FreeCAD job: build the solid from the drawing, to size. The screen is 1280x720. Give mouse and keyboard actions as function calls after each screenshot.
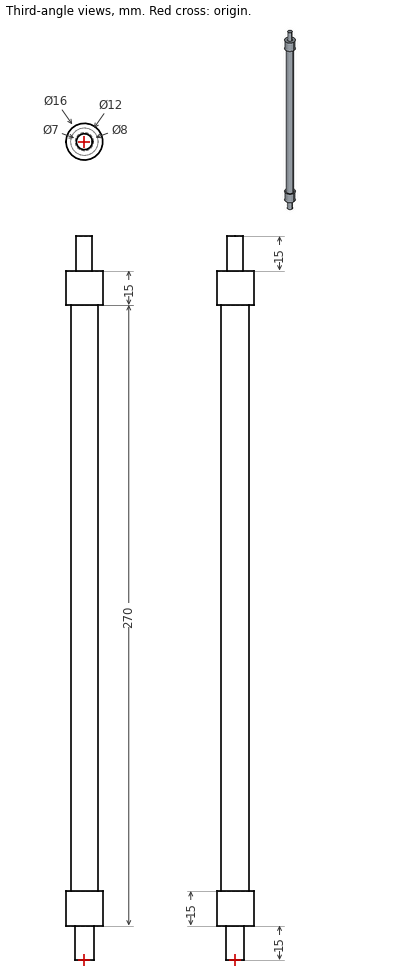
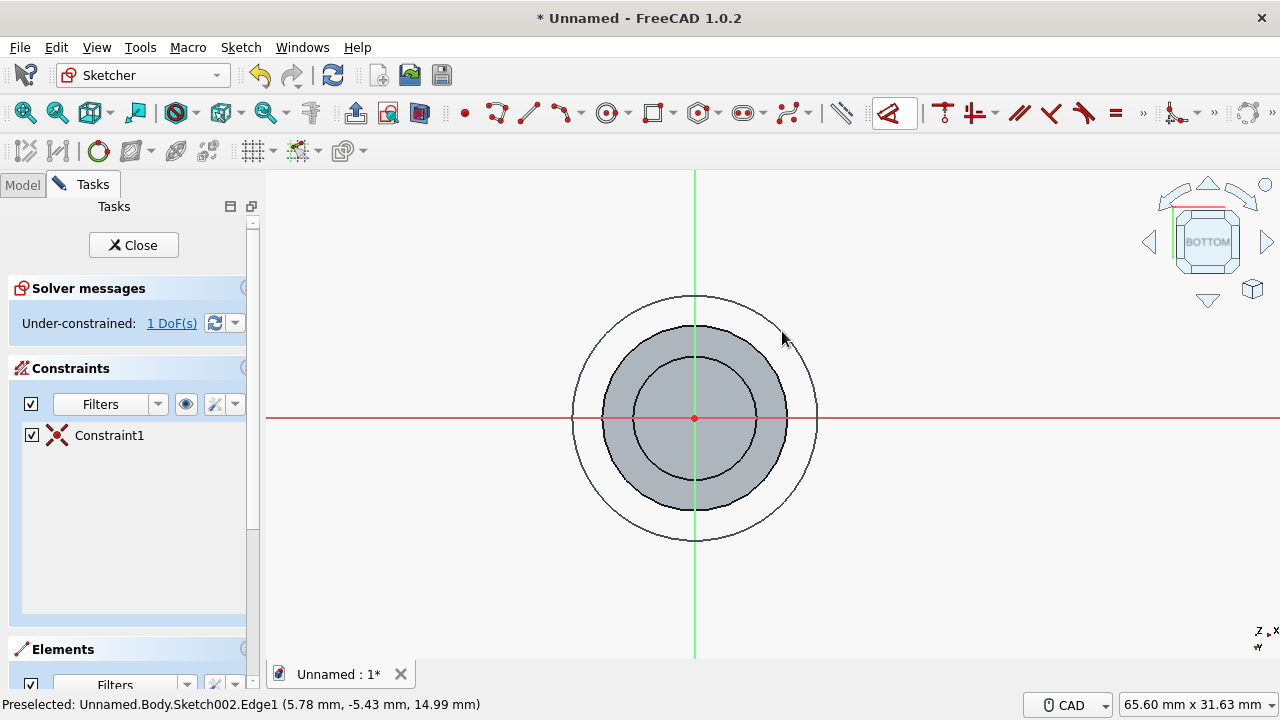
click(781, 331)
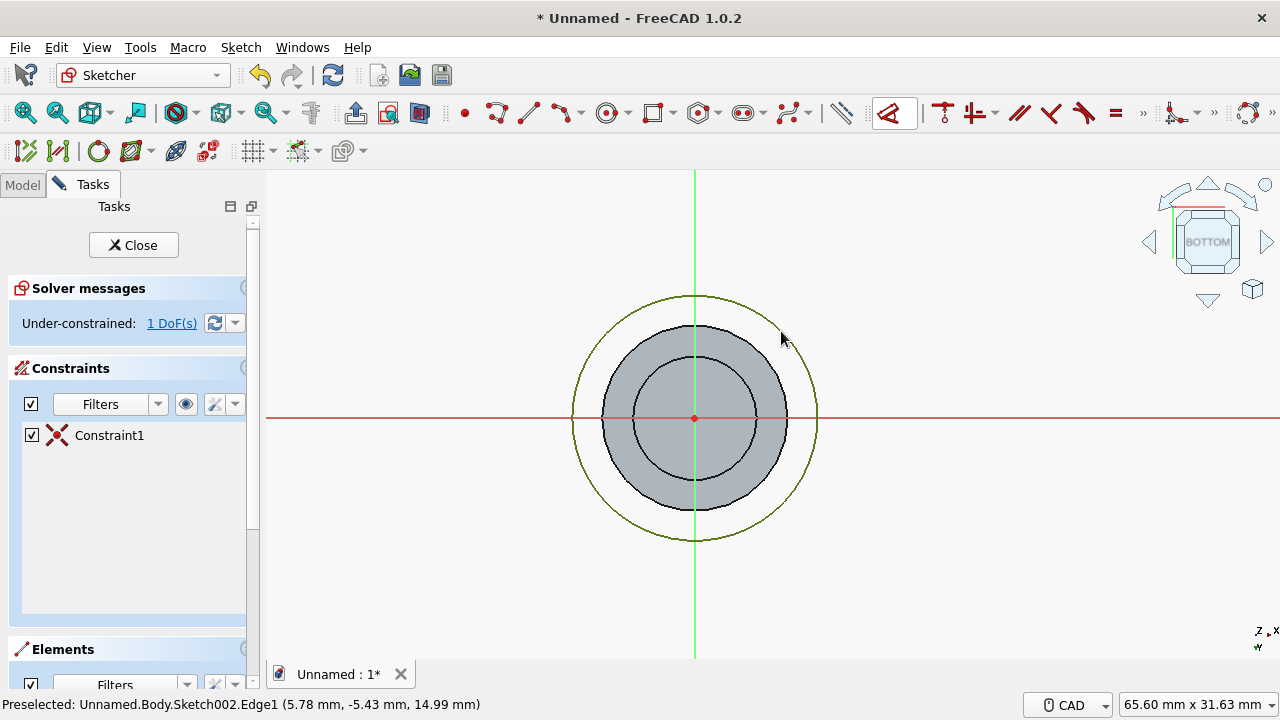
click(912, 114)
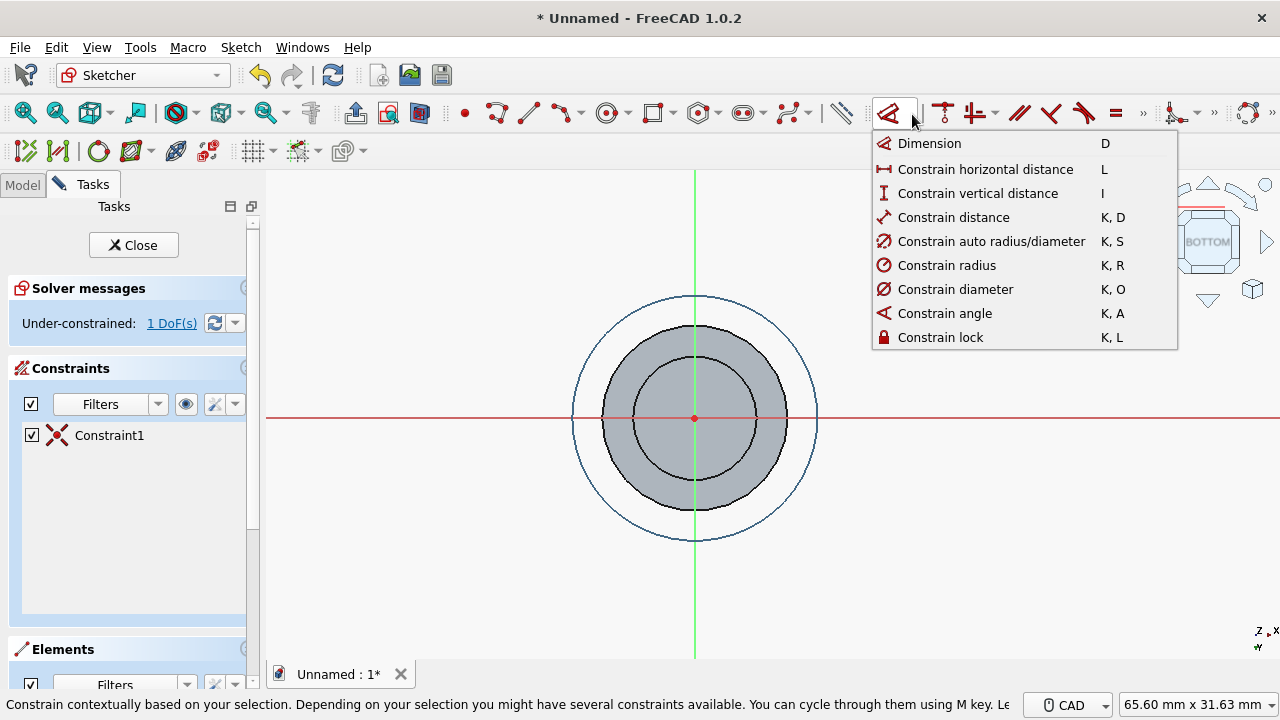
click(1025, 289)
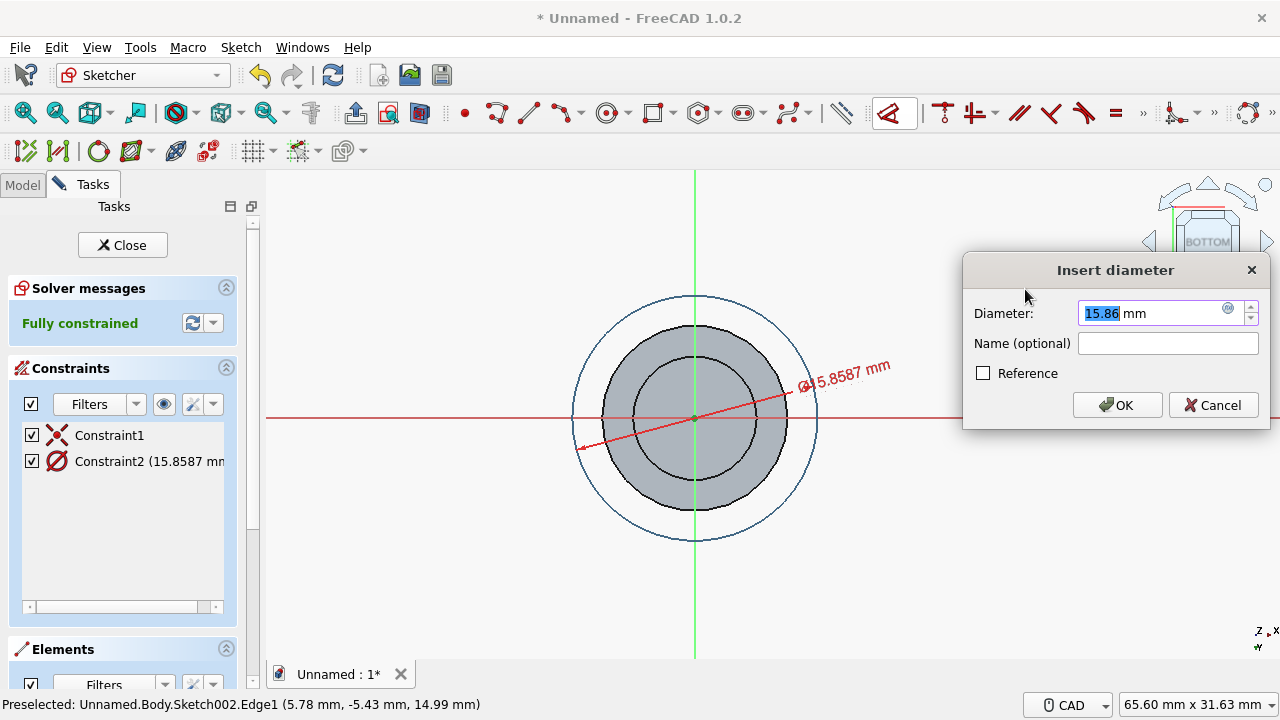
text(16)
key(Return)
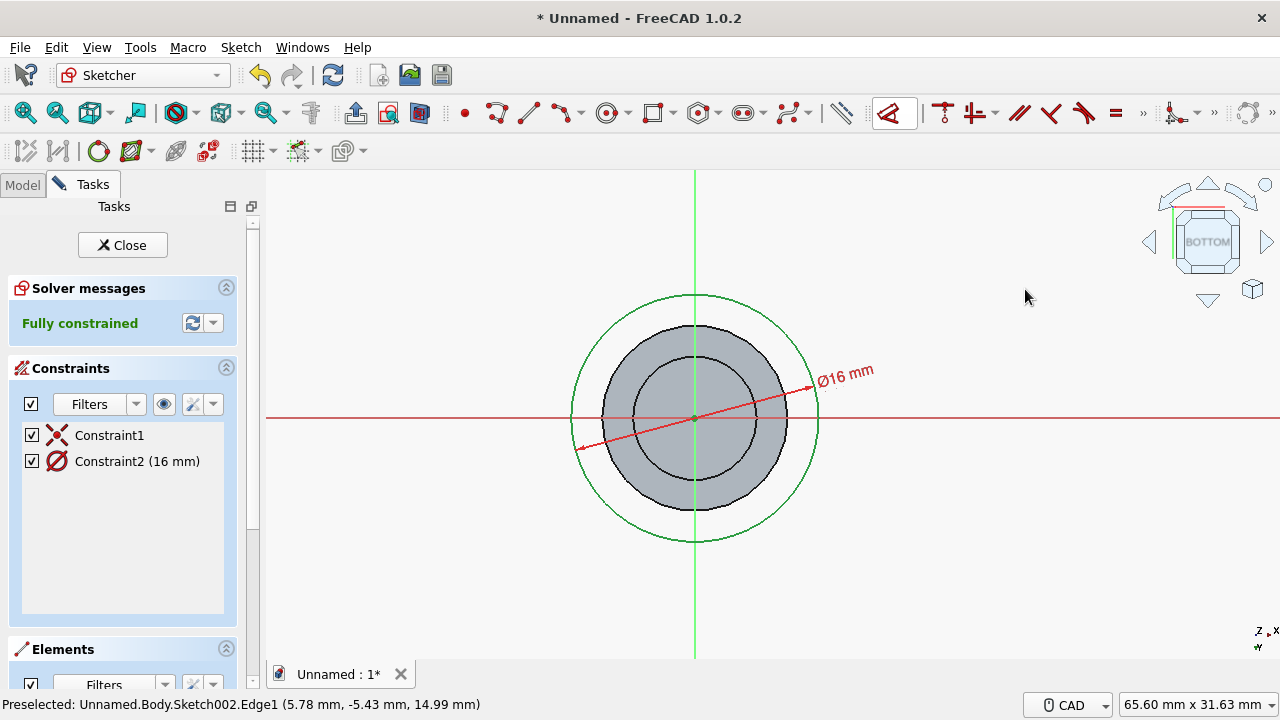
click(123, 245)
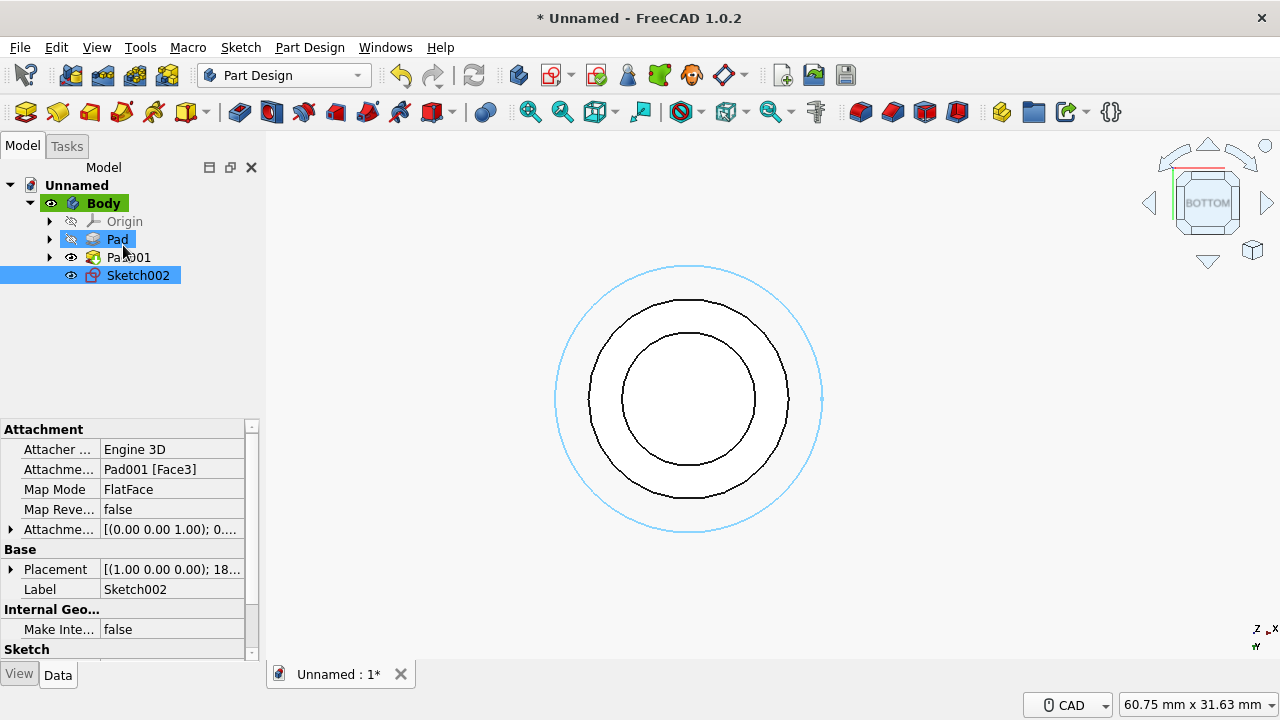
click(26, 112)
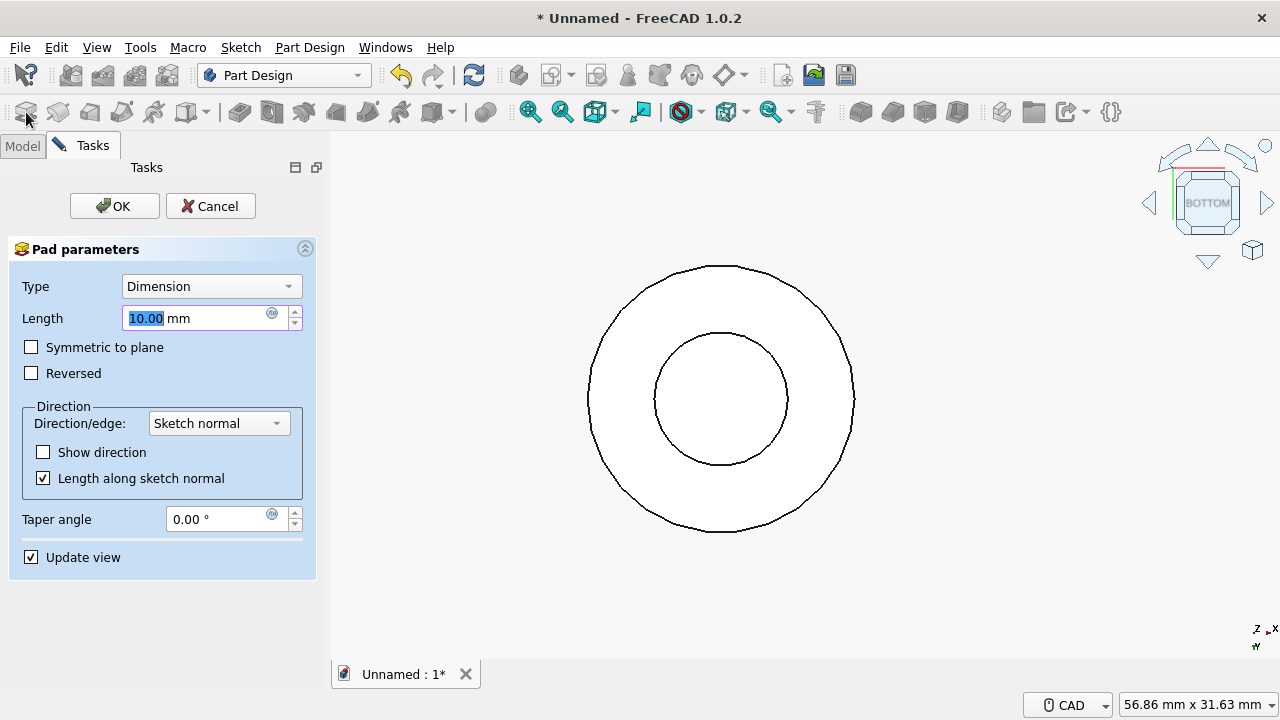
text(15)
key(Tab)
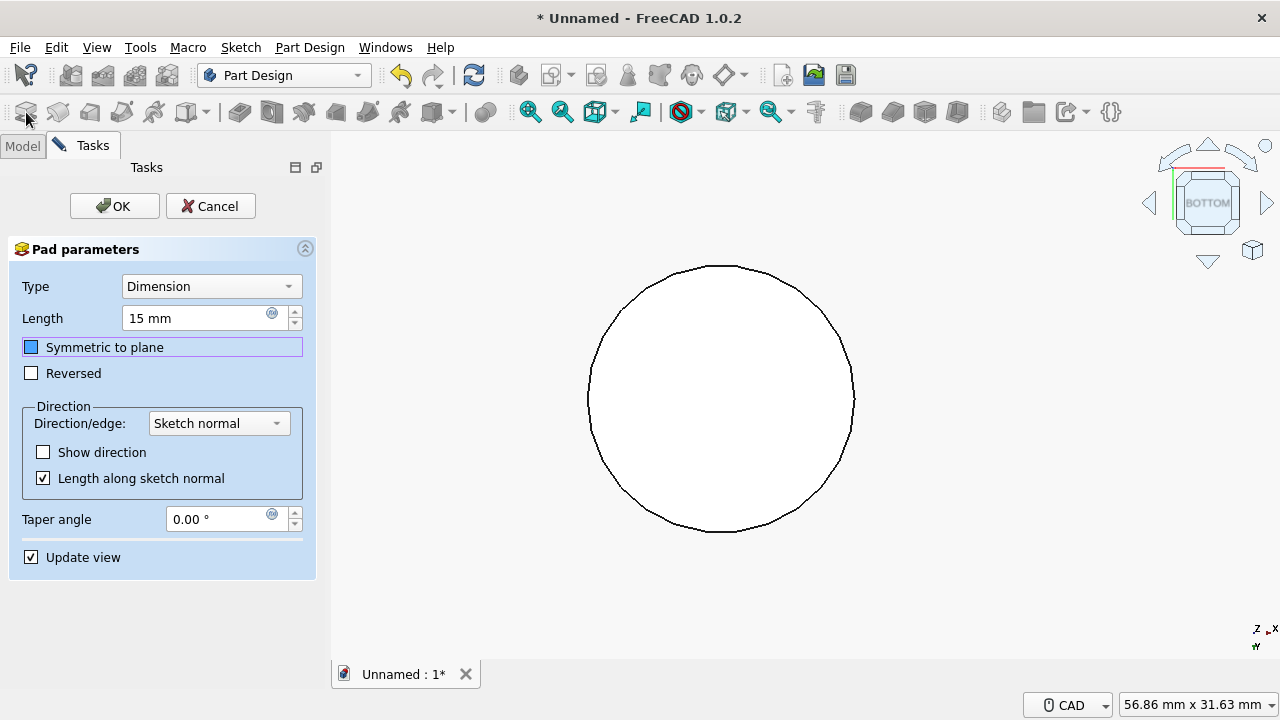
click(30, 373)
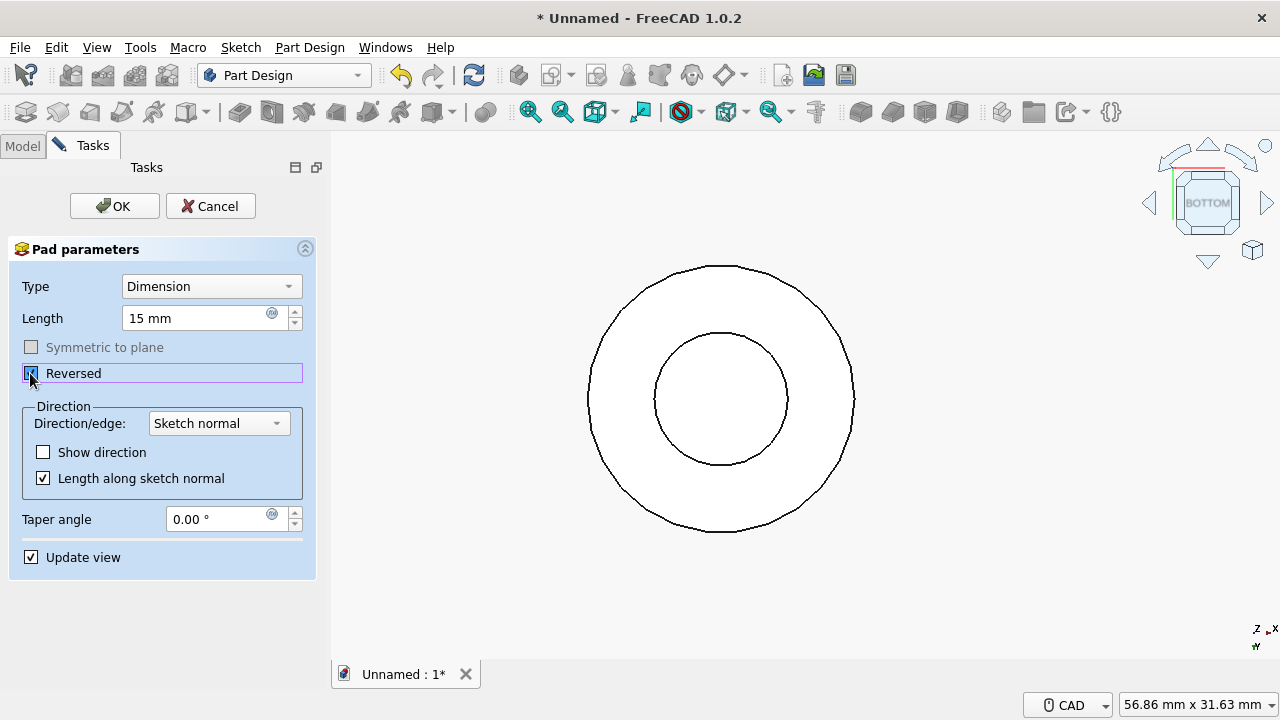
click(115, 206)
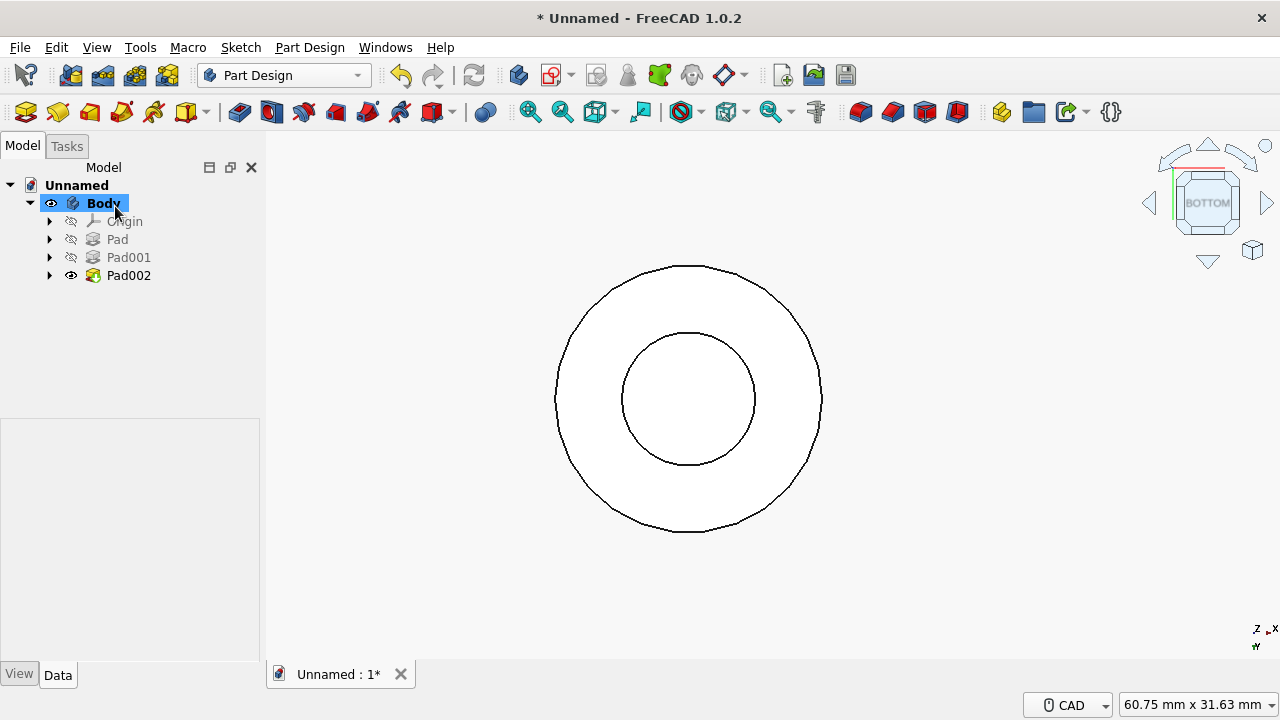
key(0)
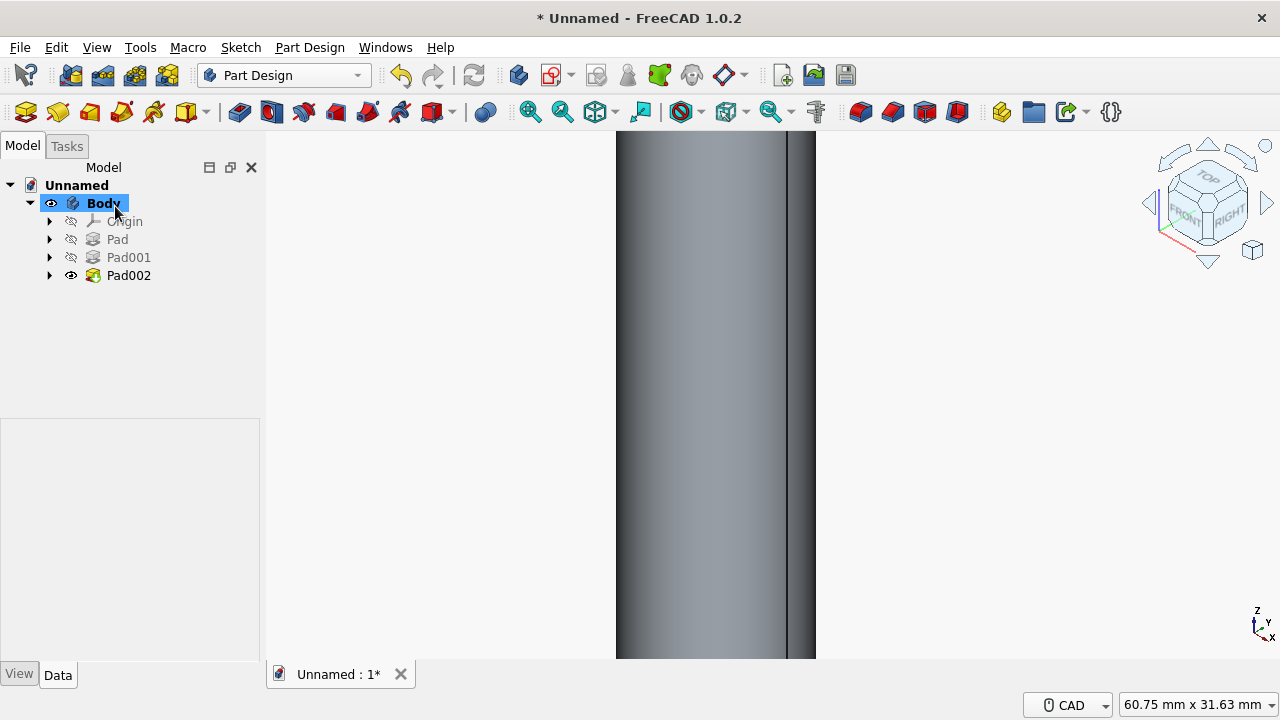
click(532, 112)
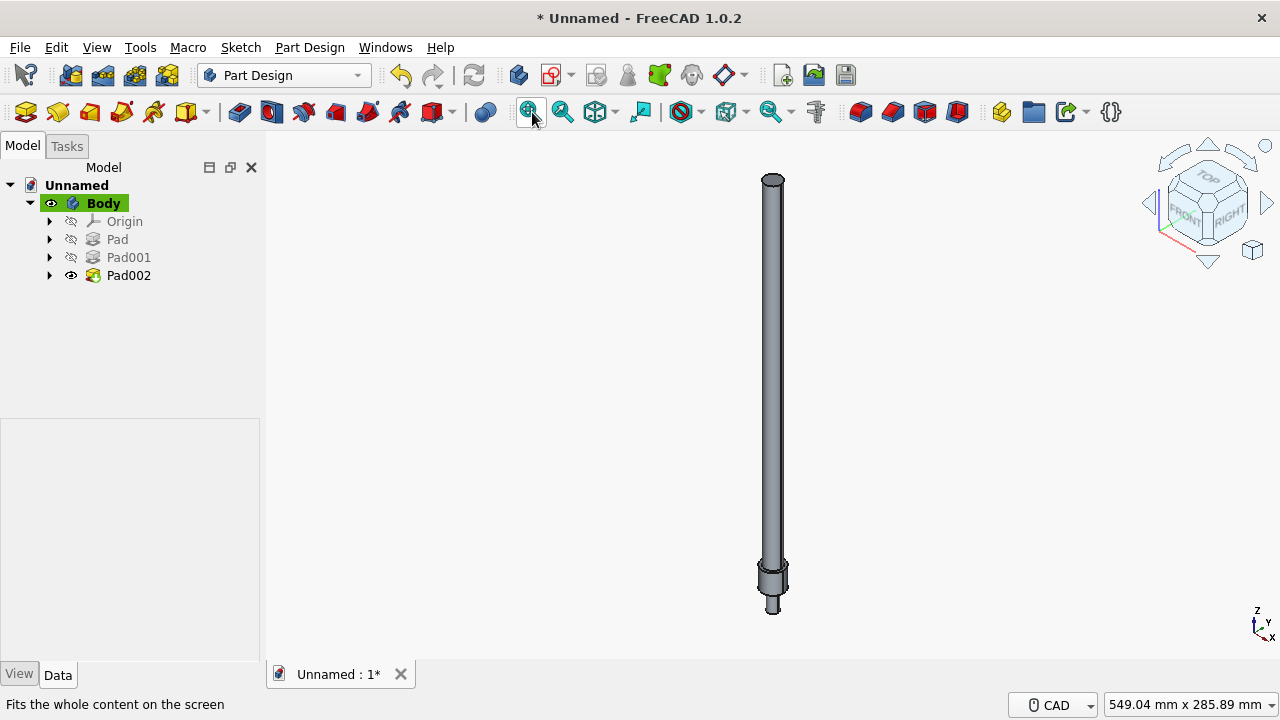
key(2)